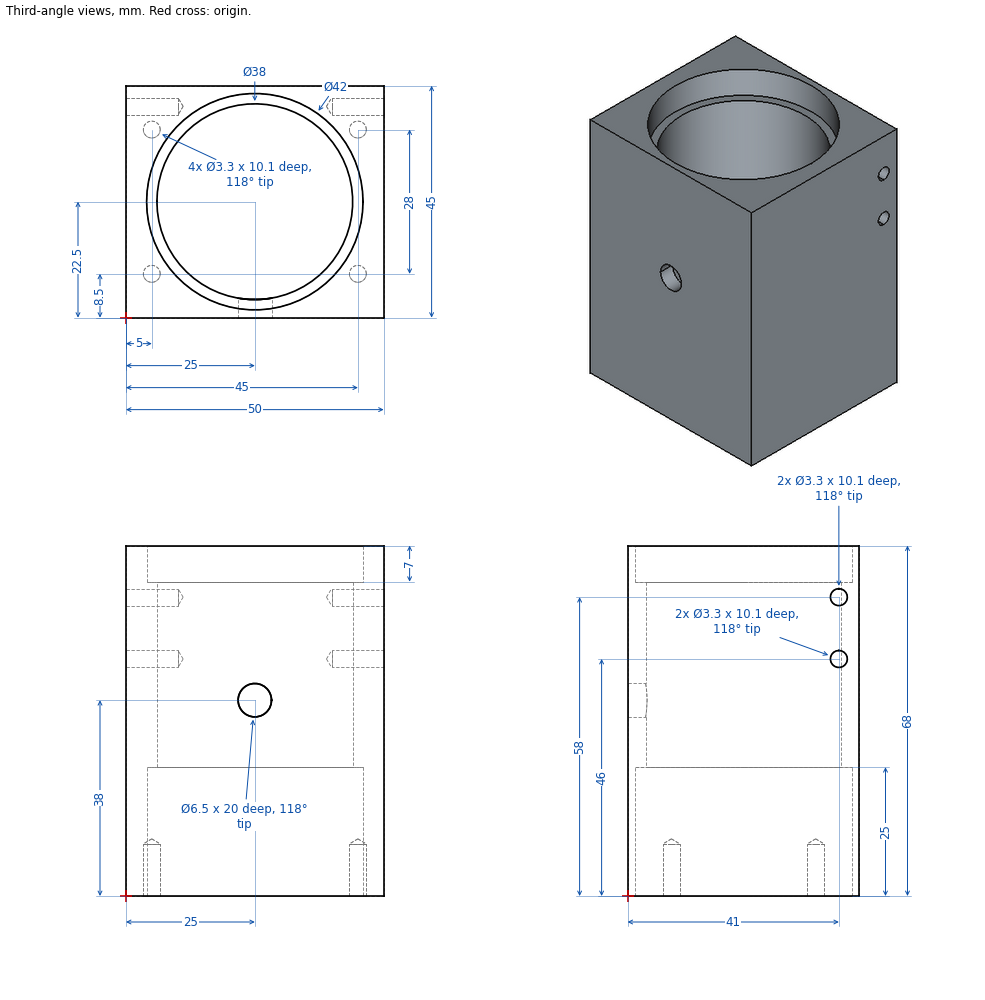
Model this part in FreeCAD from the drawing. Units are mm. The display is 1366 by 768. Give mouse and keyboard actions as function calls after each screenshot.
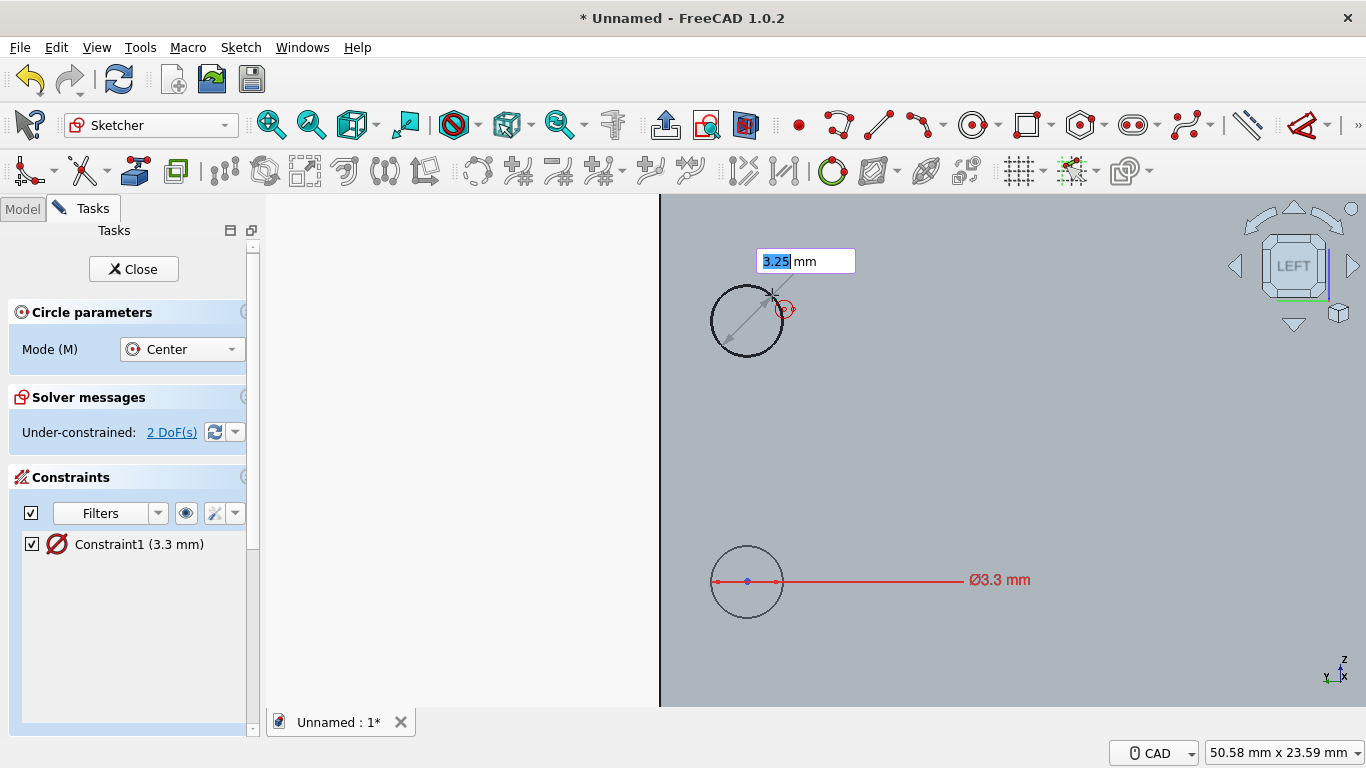
text(3.3)
key(Return)
key(Escape)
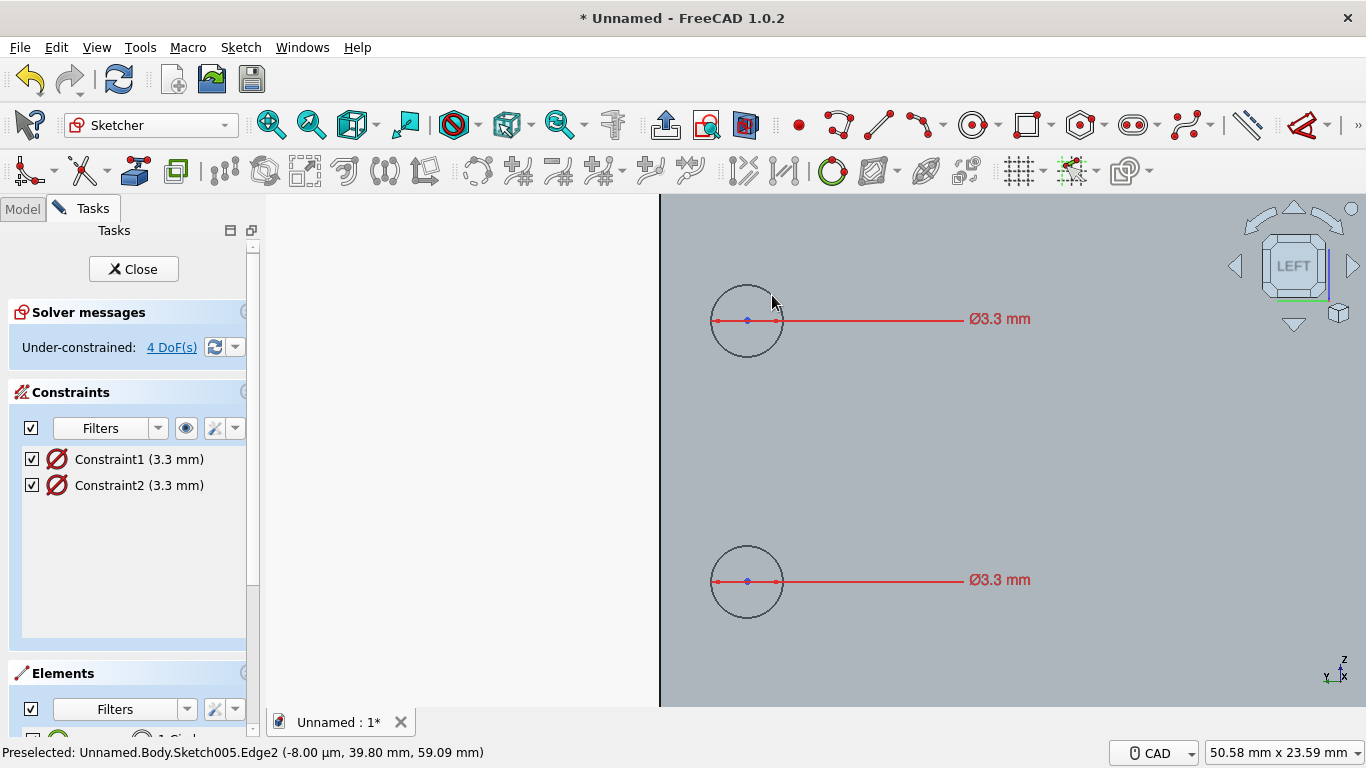
click(747, 582)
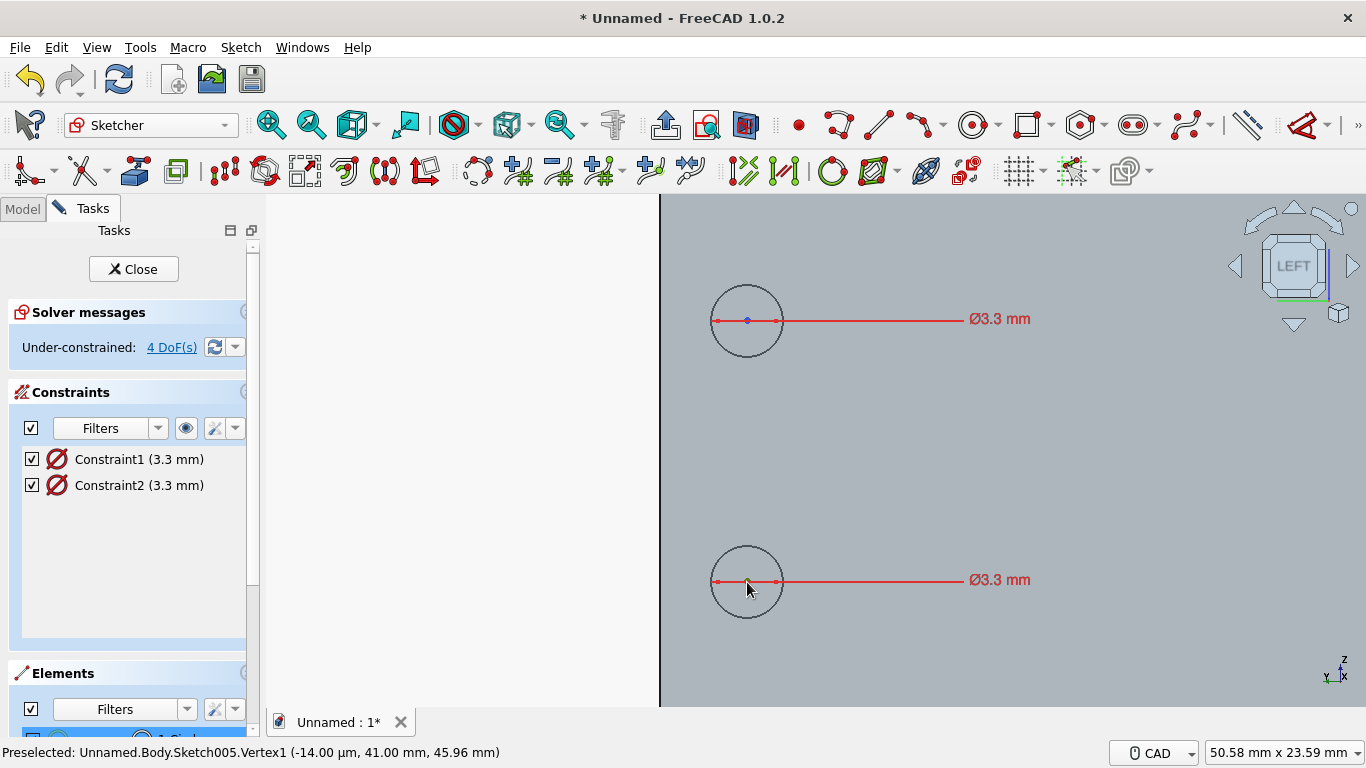
click(747, 321)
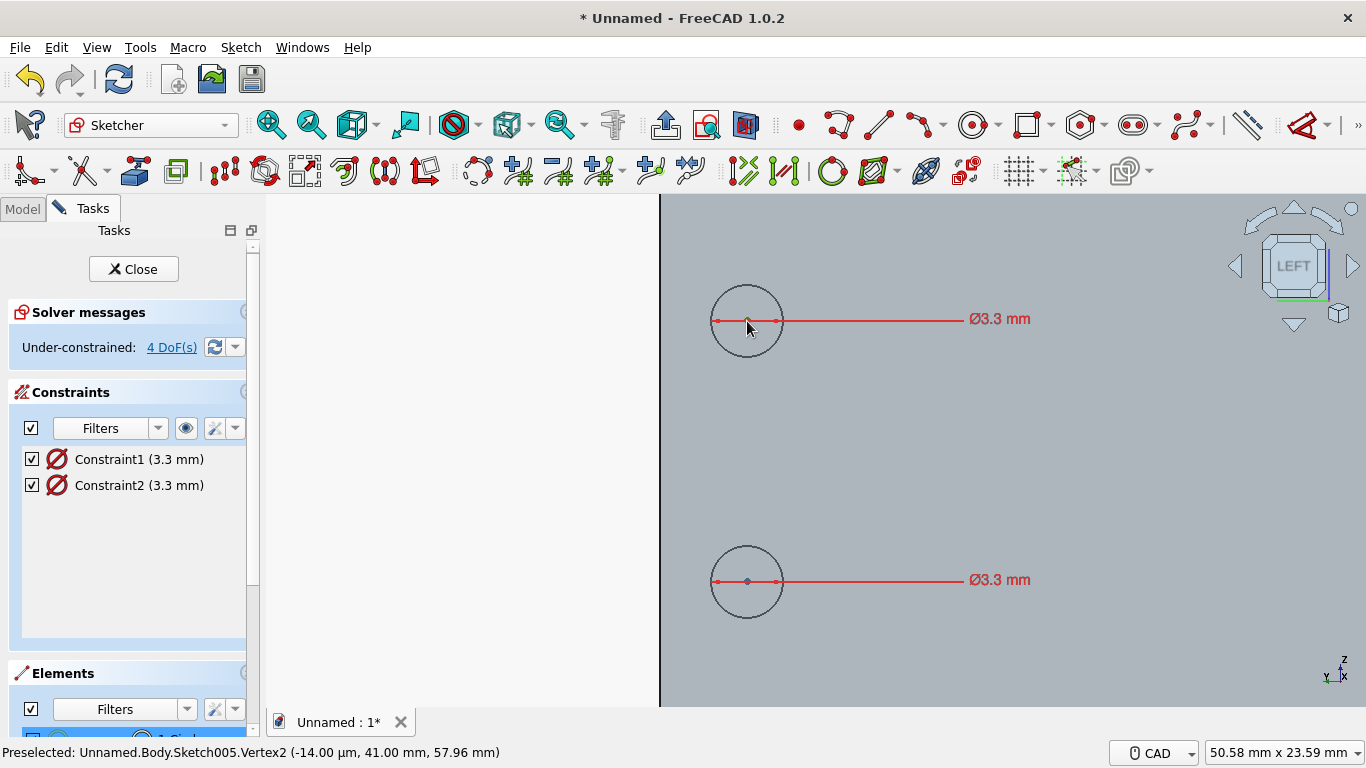
key(v)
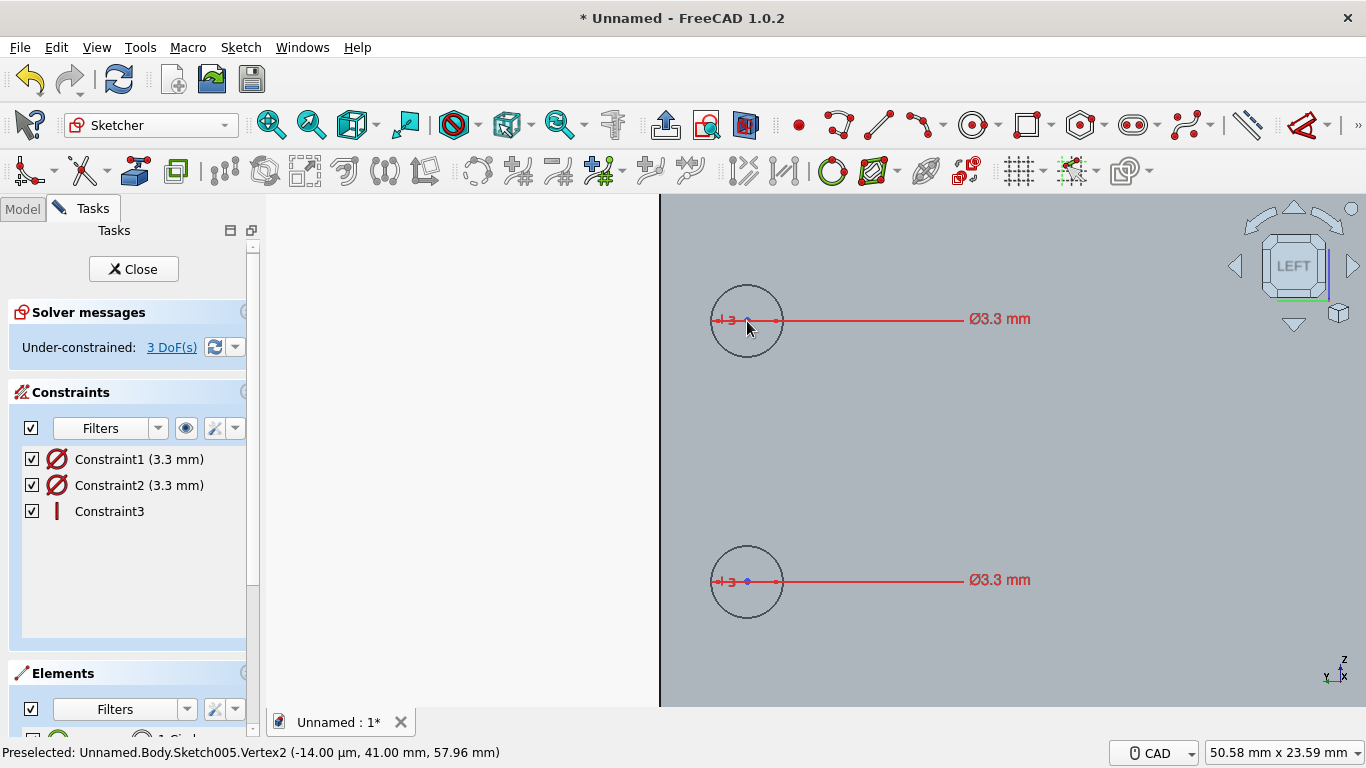
click(1302, 126)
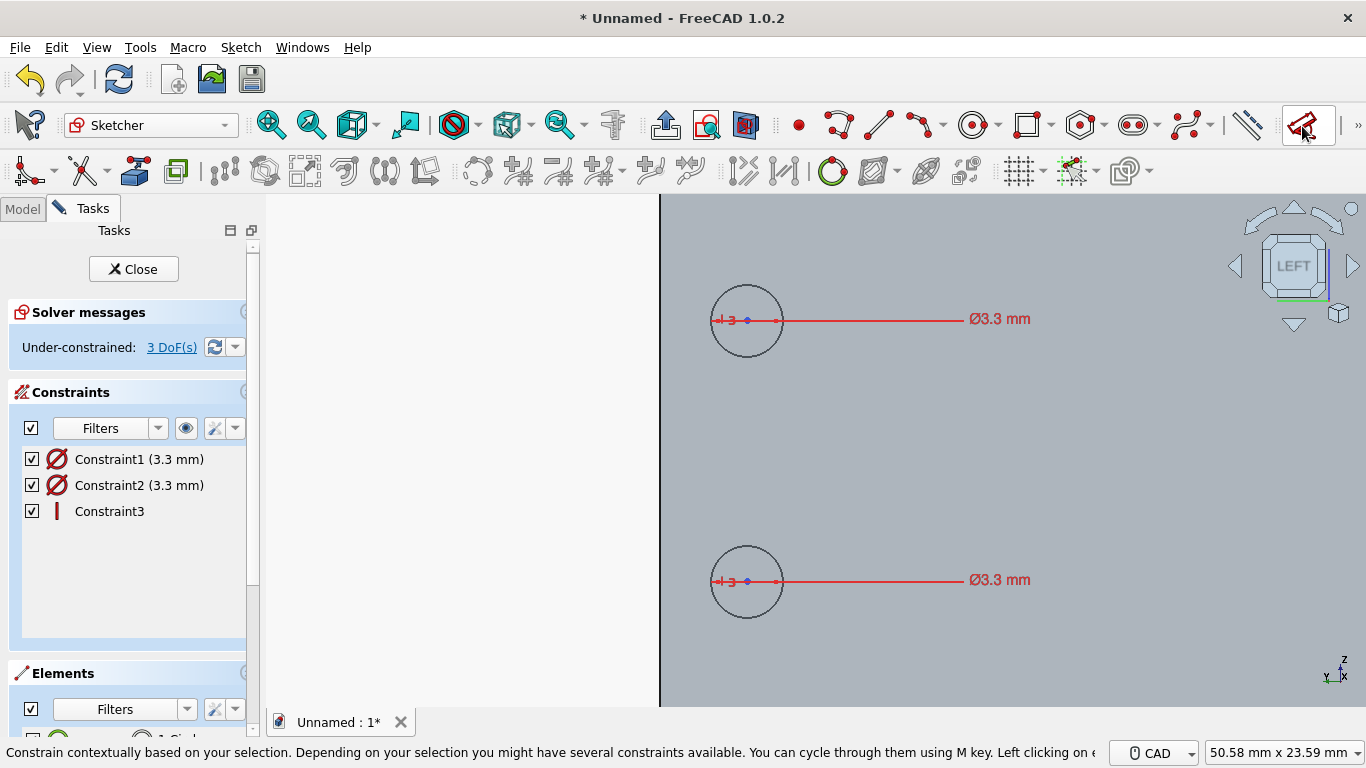
click(747, 582)
click(974, 548)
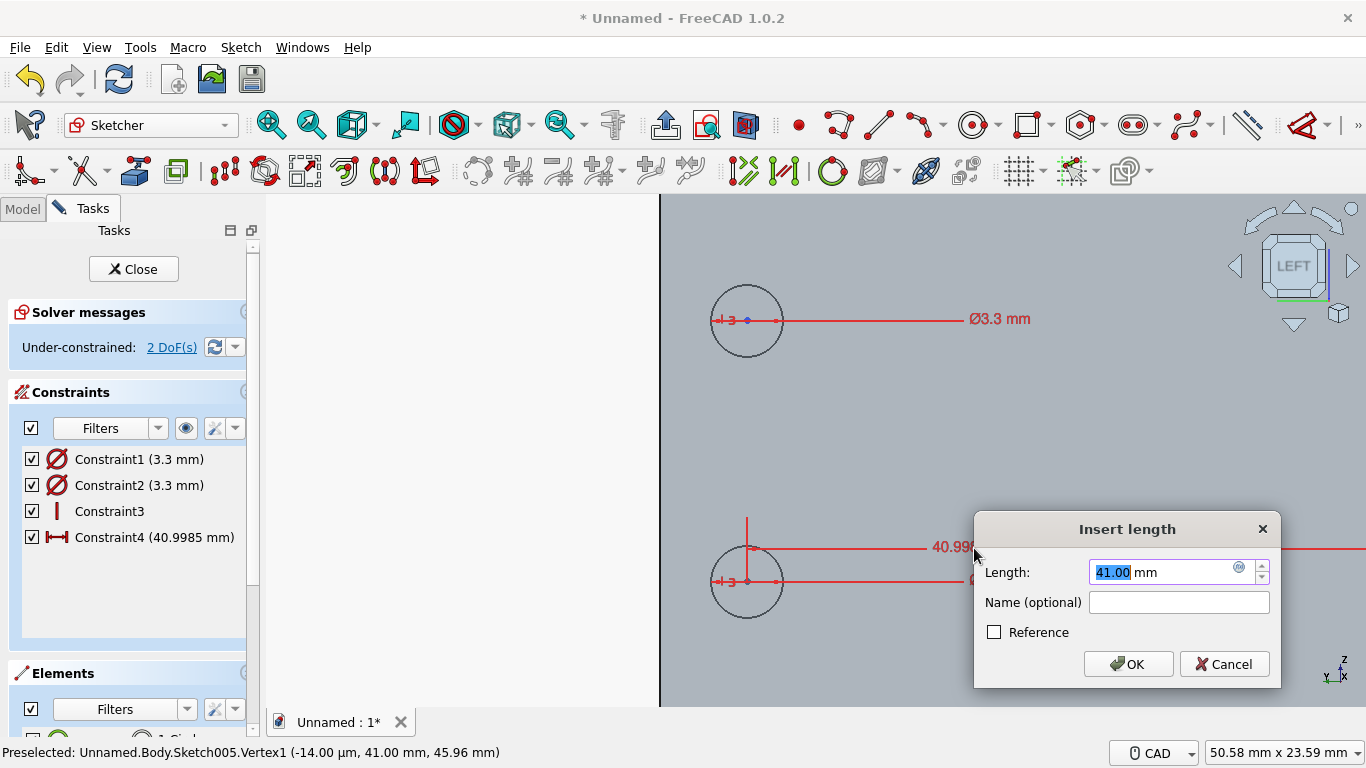
text(41)
key(Return)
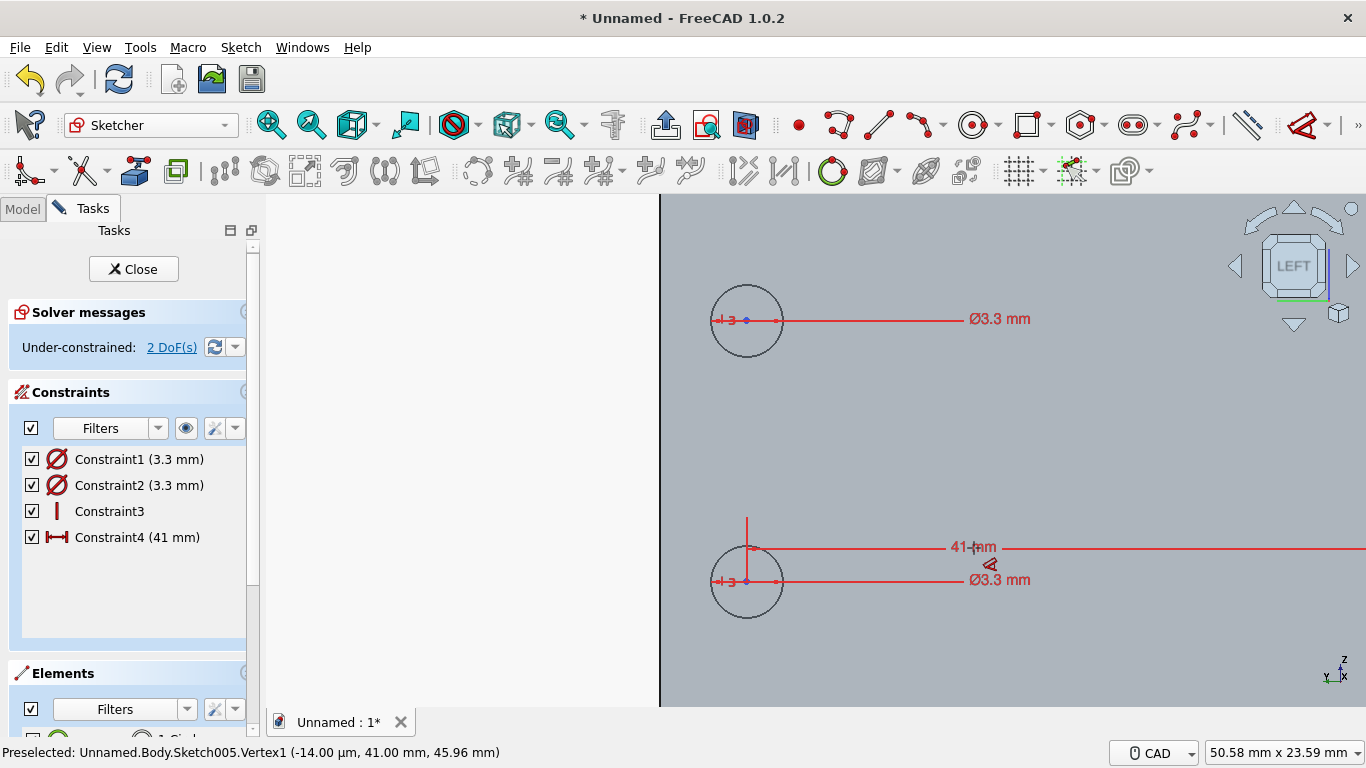
click(747, 582)
click(713, 631)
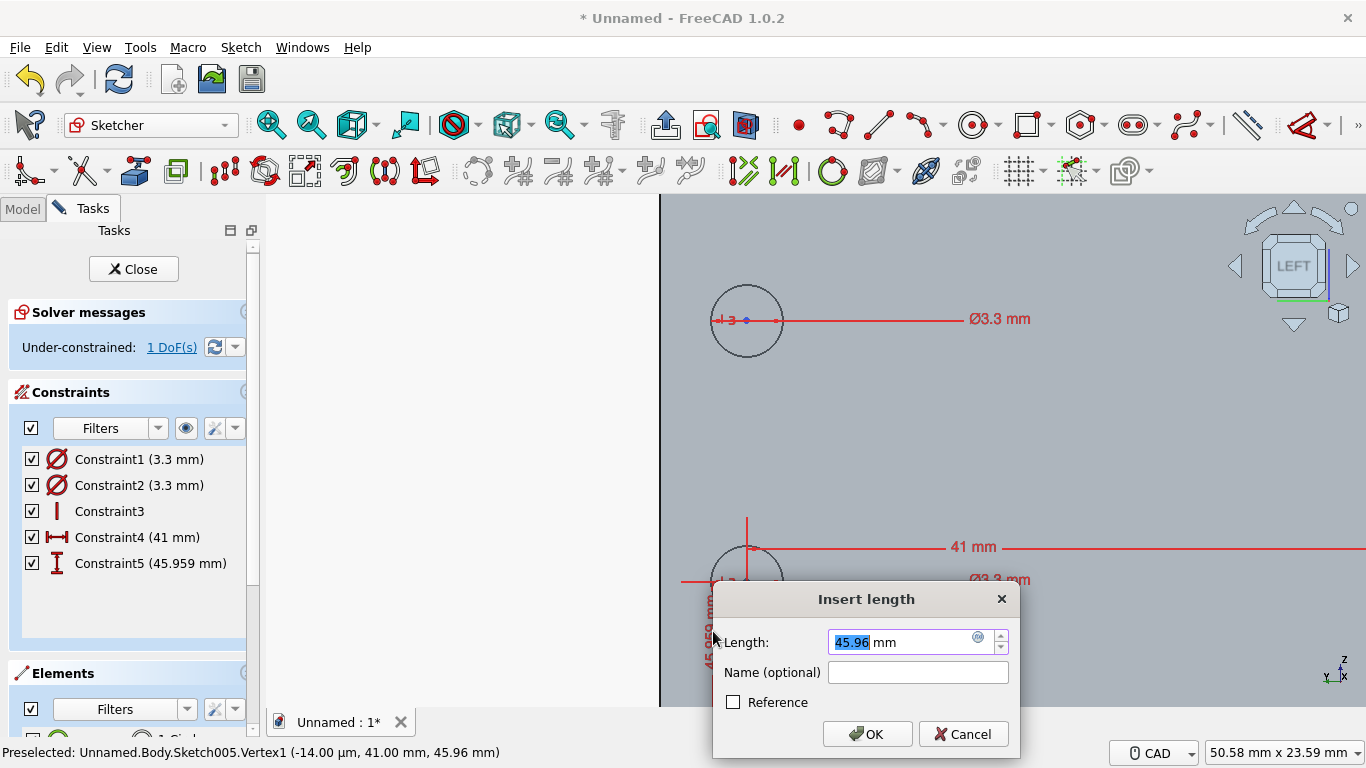
text(46)
key(Return)